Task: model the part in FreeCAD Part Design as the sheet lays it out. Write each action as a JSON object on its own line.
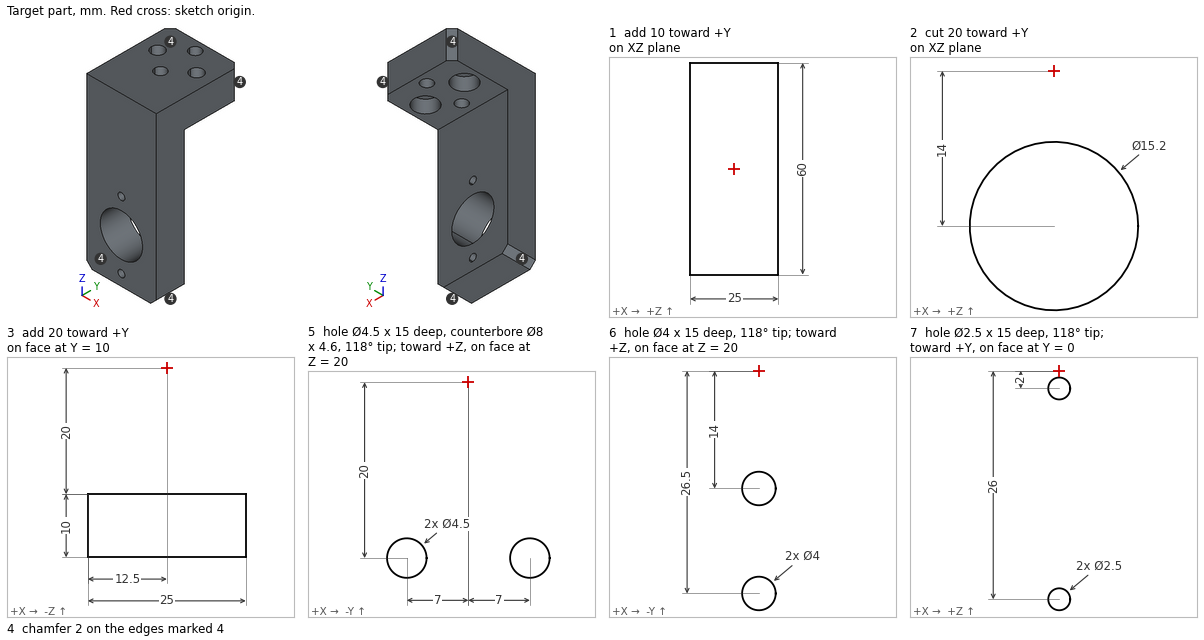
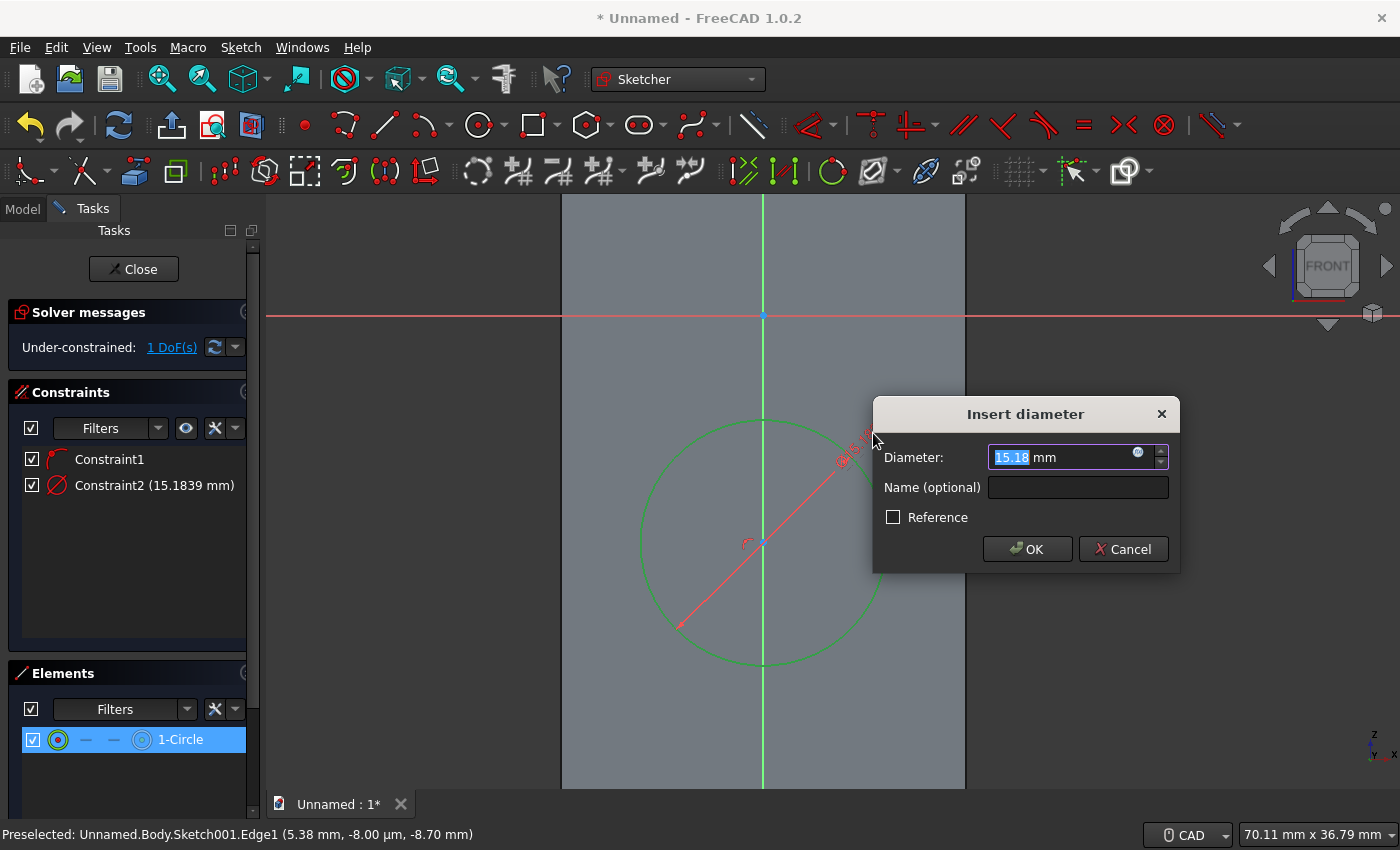
{"action": "type", "text": "15.2"}
{"action": "key", "text": "Return"}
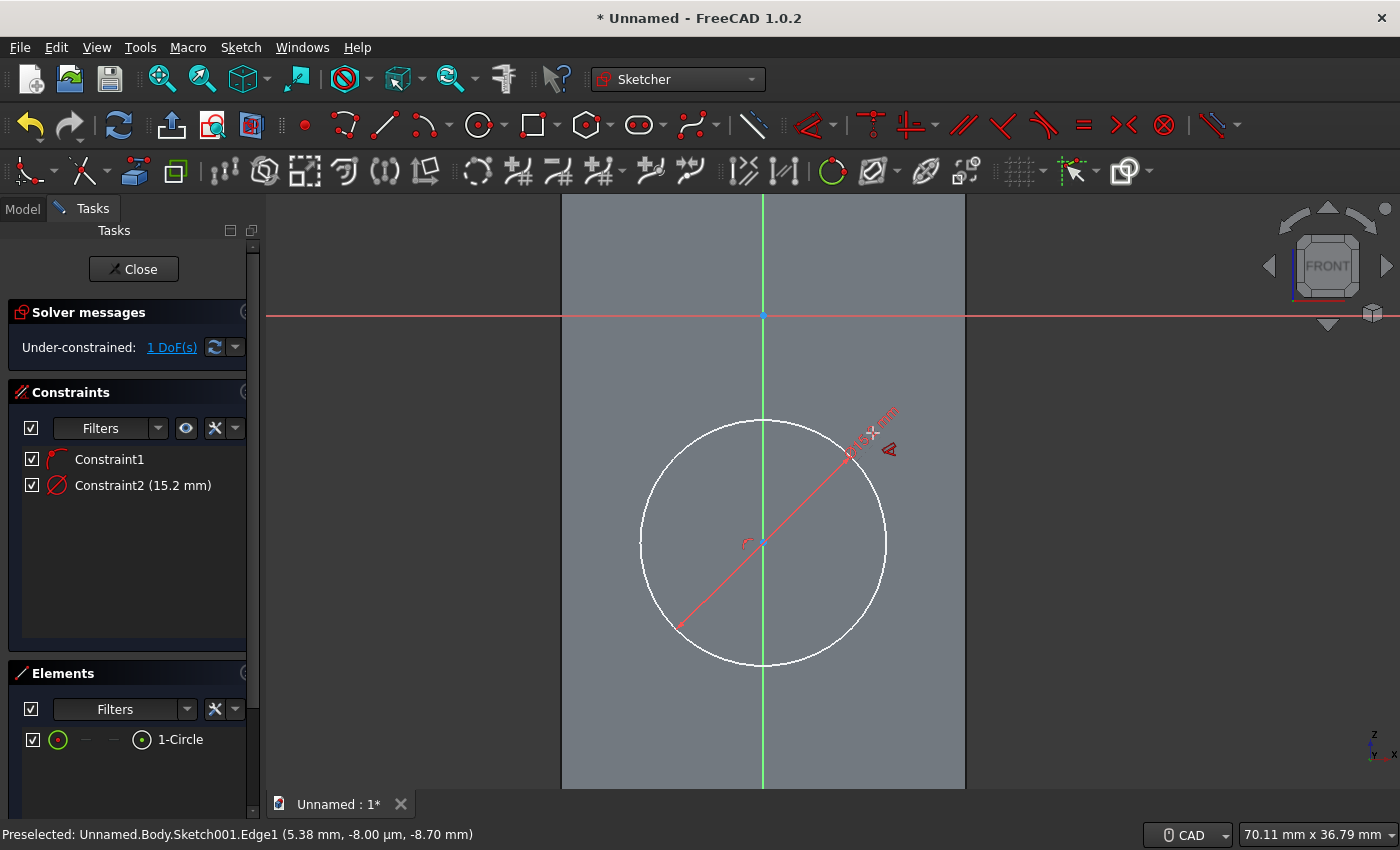
{"action": "left_click", "coordinate": [763, 543]}
{"action": "left_click", "coordinate": [797, 377]}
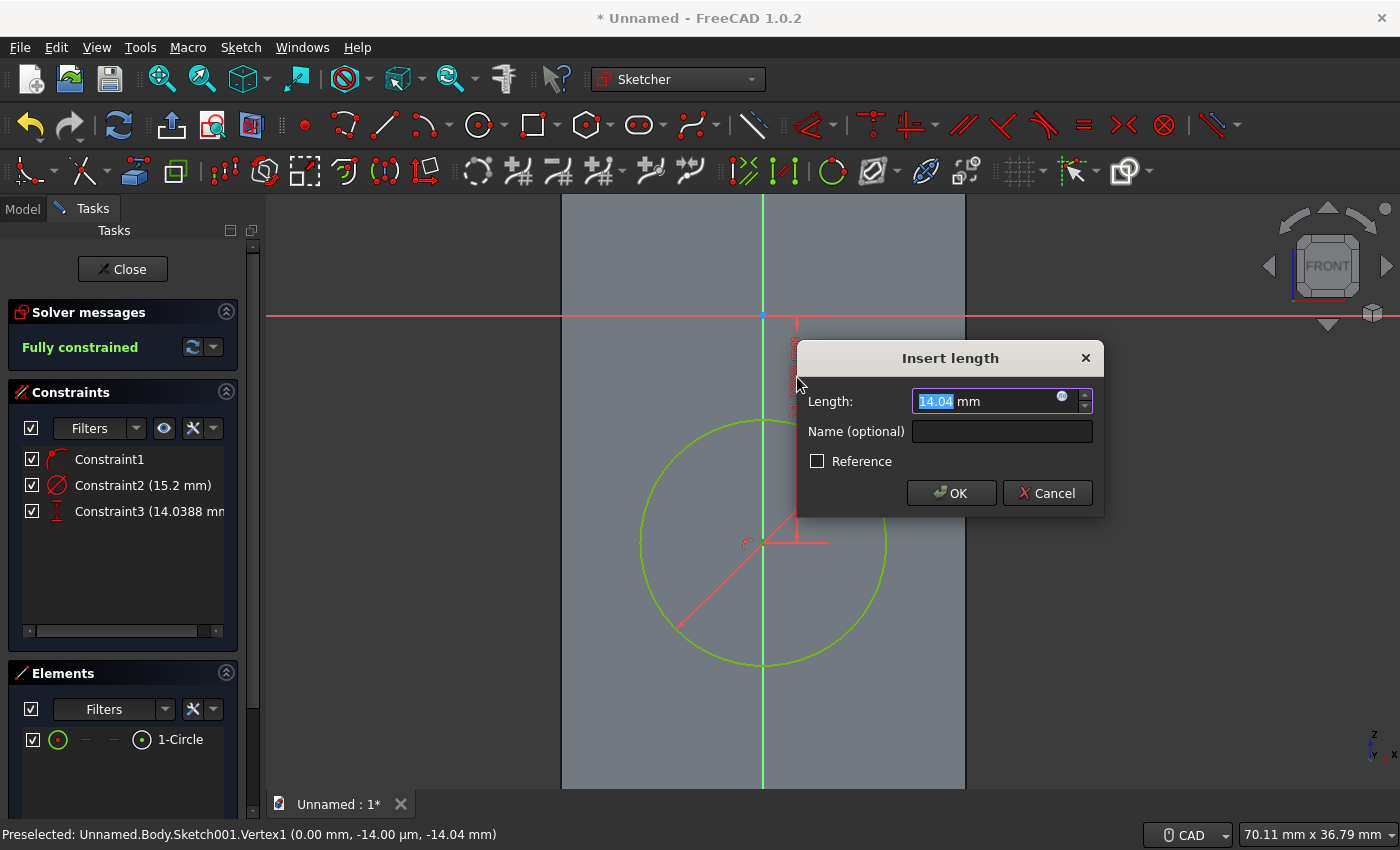
{"action": "type", "text": "14"}
{"action": "key", "text": "Return"}
{"action": "key", "text": "Escape"}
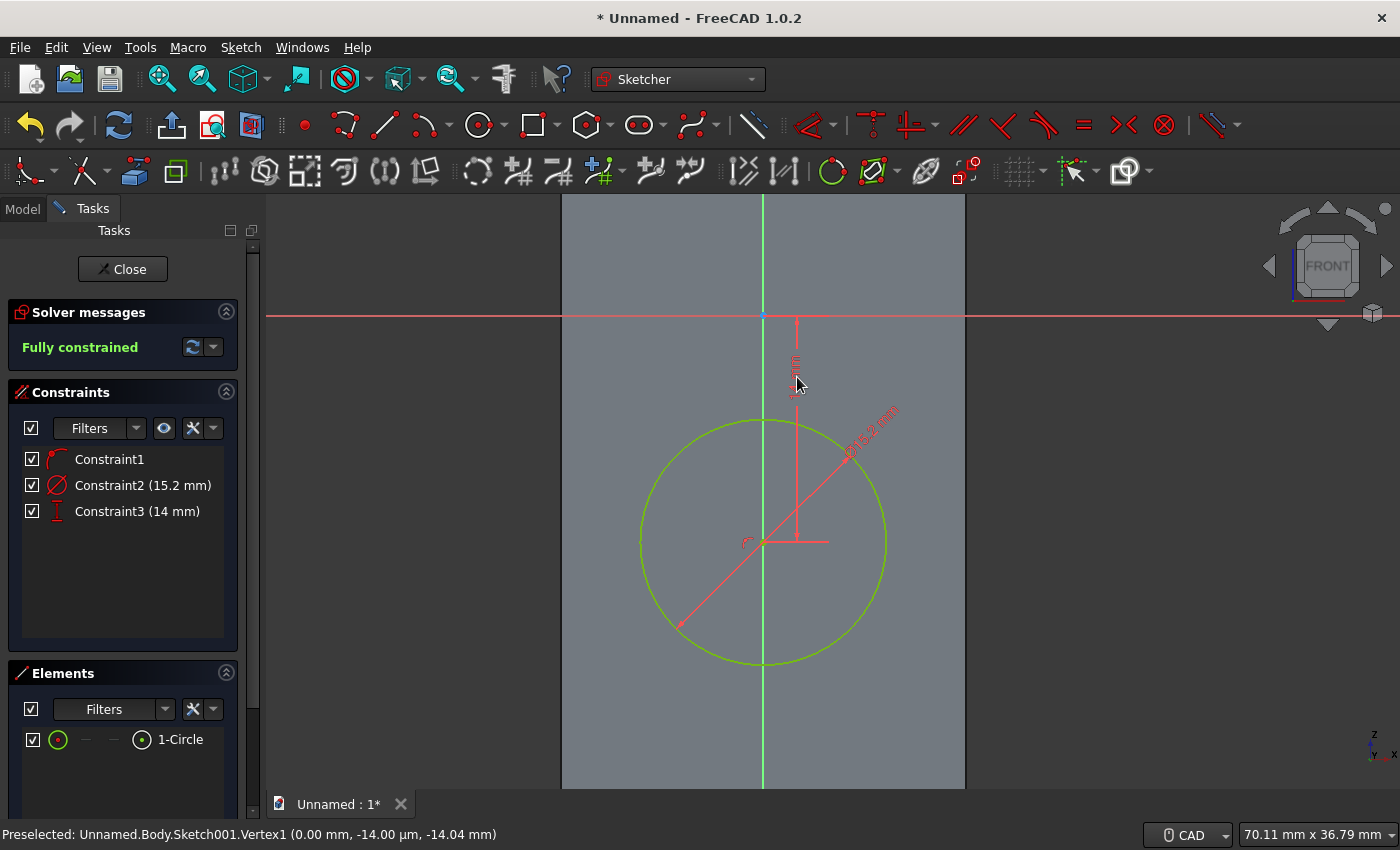
{"action": "left_click", "coordinate": [123, 269]}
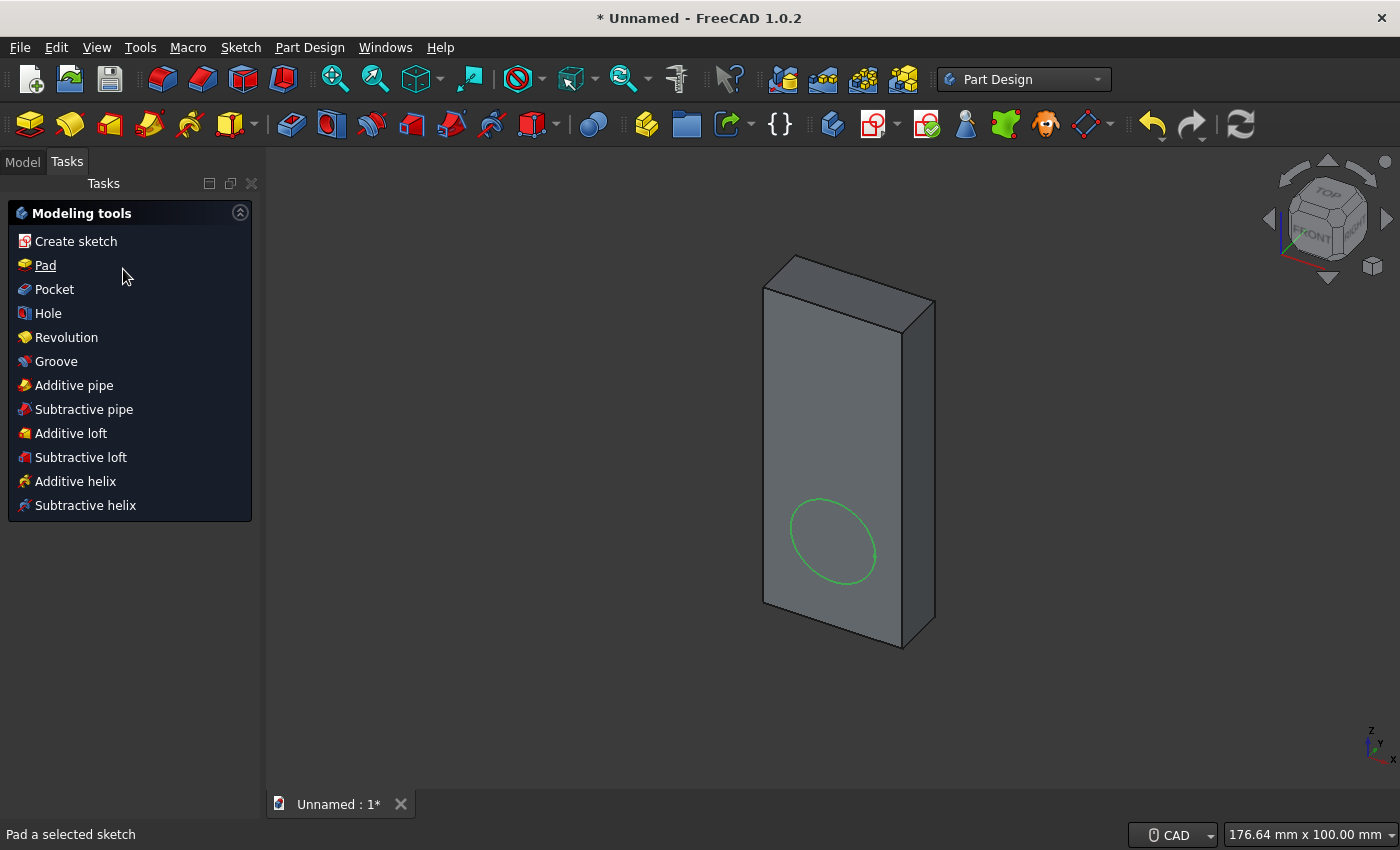
{"action": "left_click", "coordinate": [292, 124]}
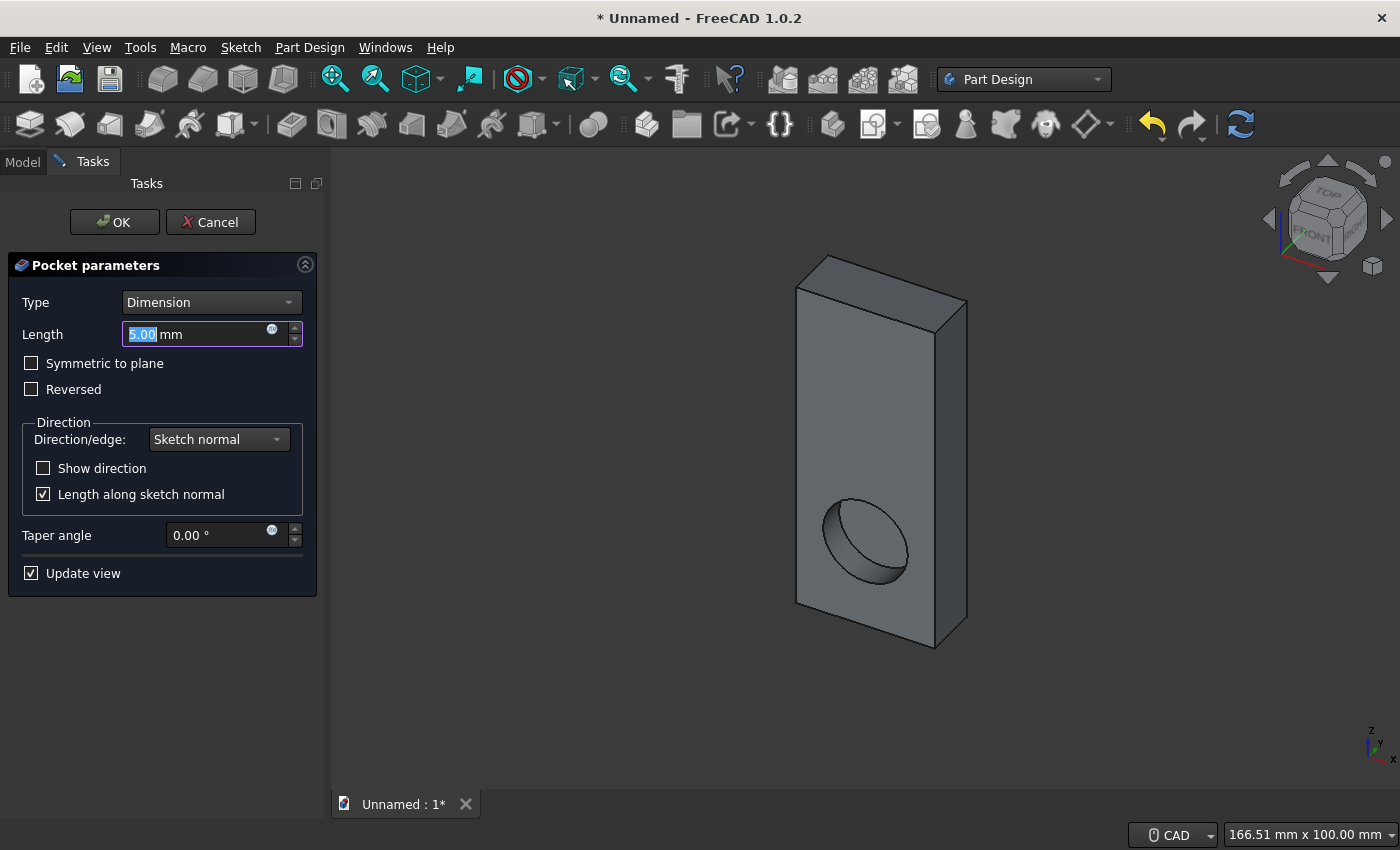
{"action": "type", "text": "20"}
{"action": "key", "text": "Tab"}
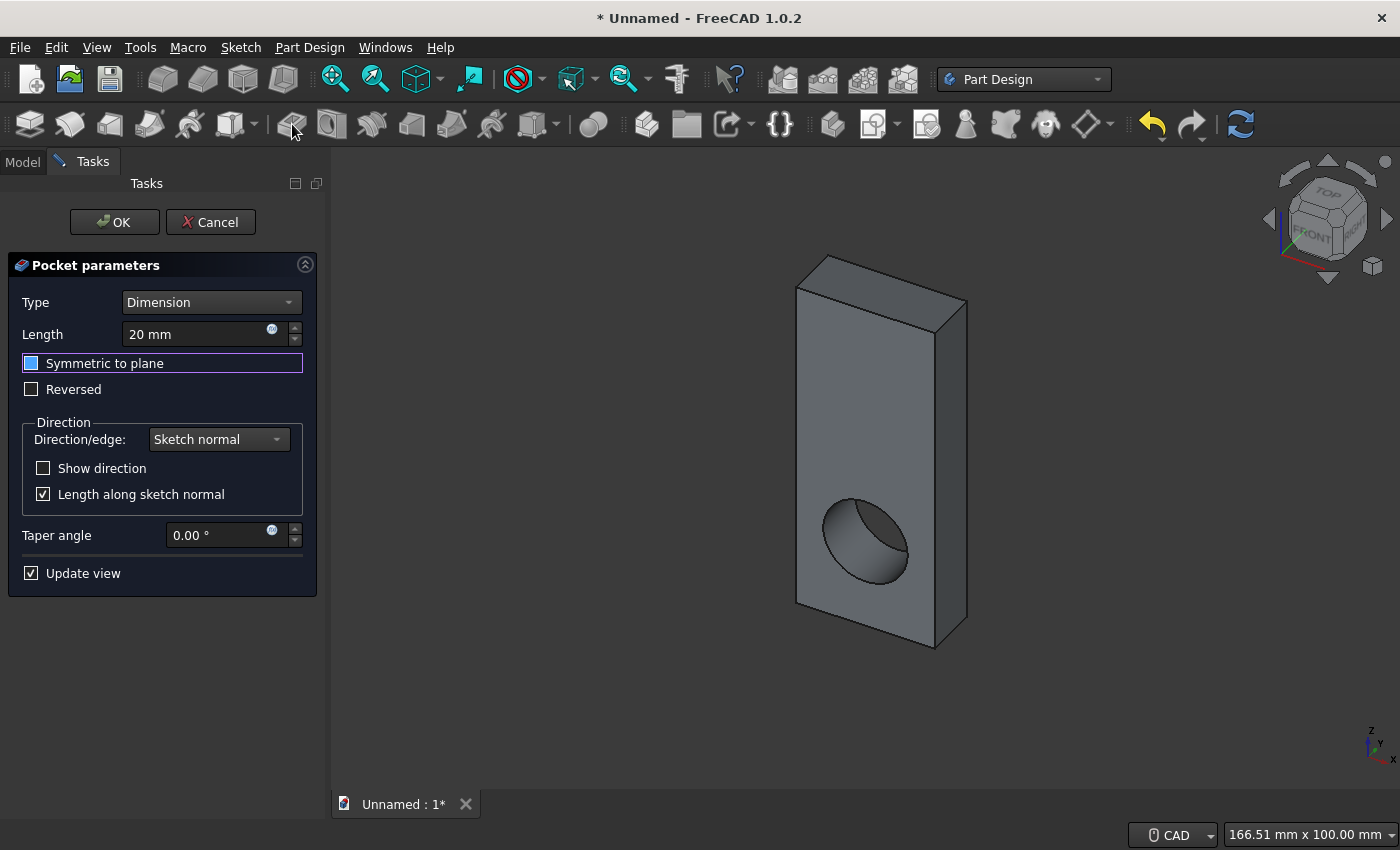
{"action": "left_click", "coordinate": [115, 222]}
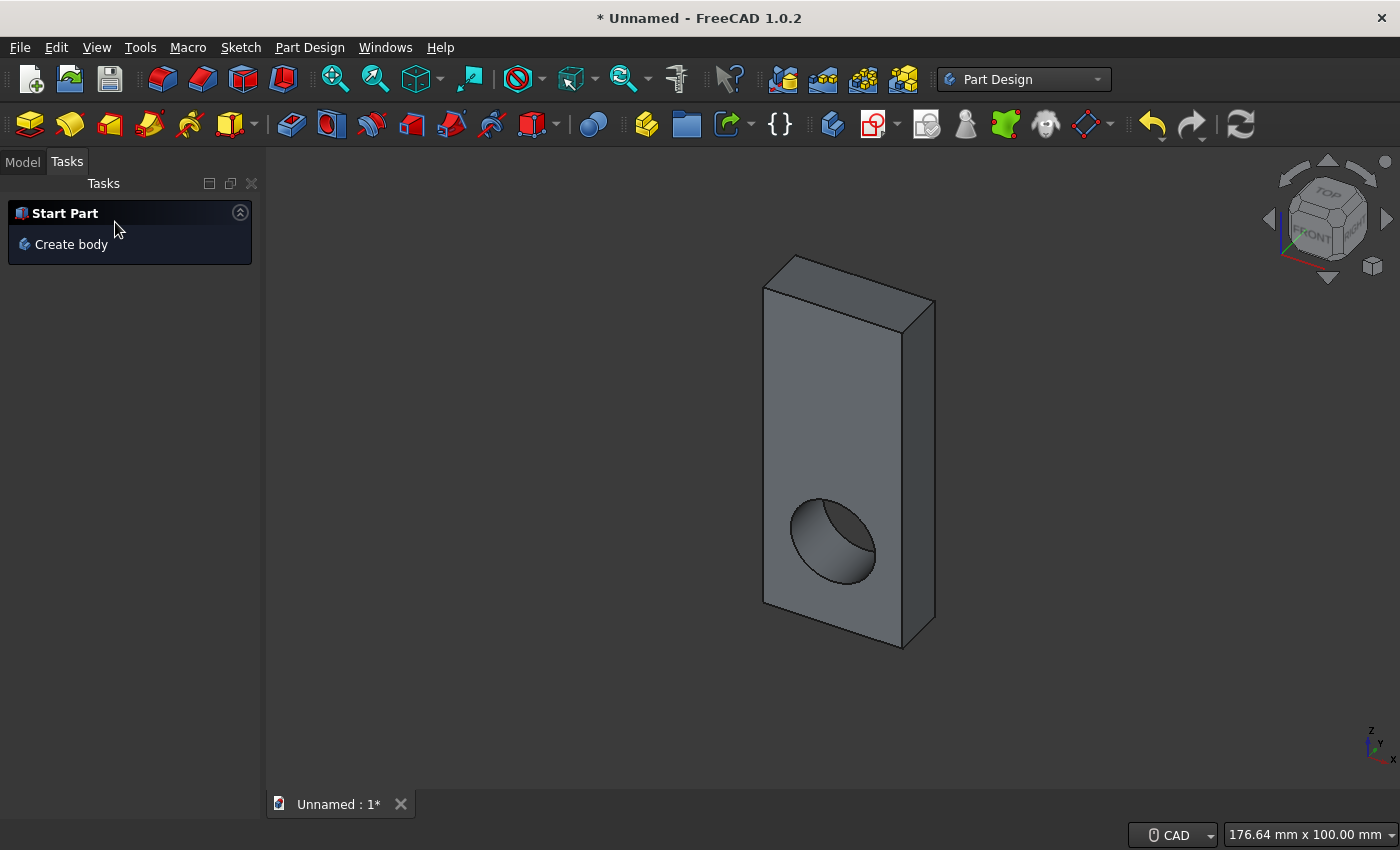
{"action": "key", "text": "4"}